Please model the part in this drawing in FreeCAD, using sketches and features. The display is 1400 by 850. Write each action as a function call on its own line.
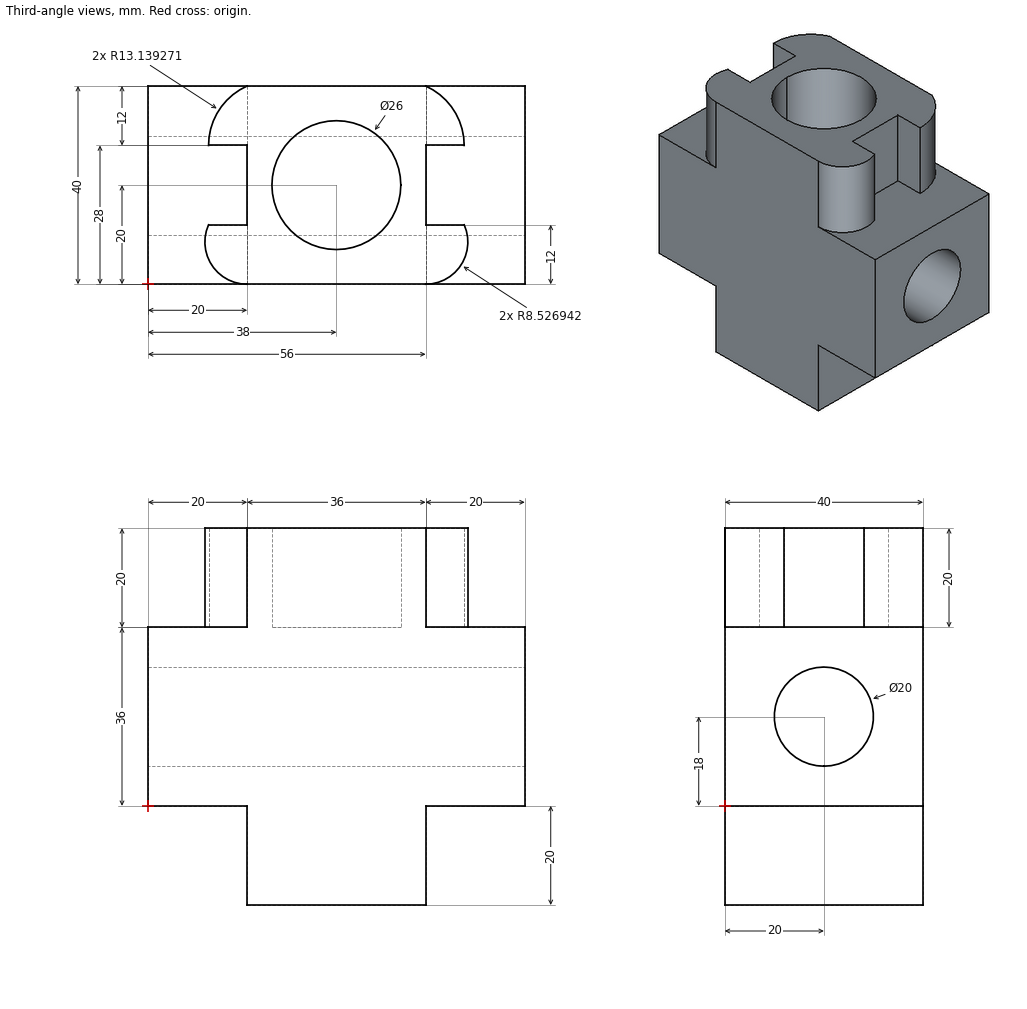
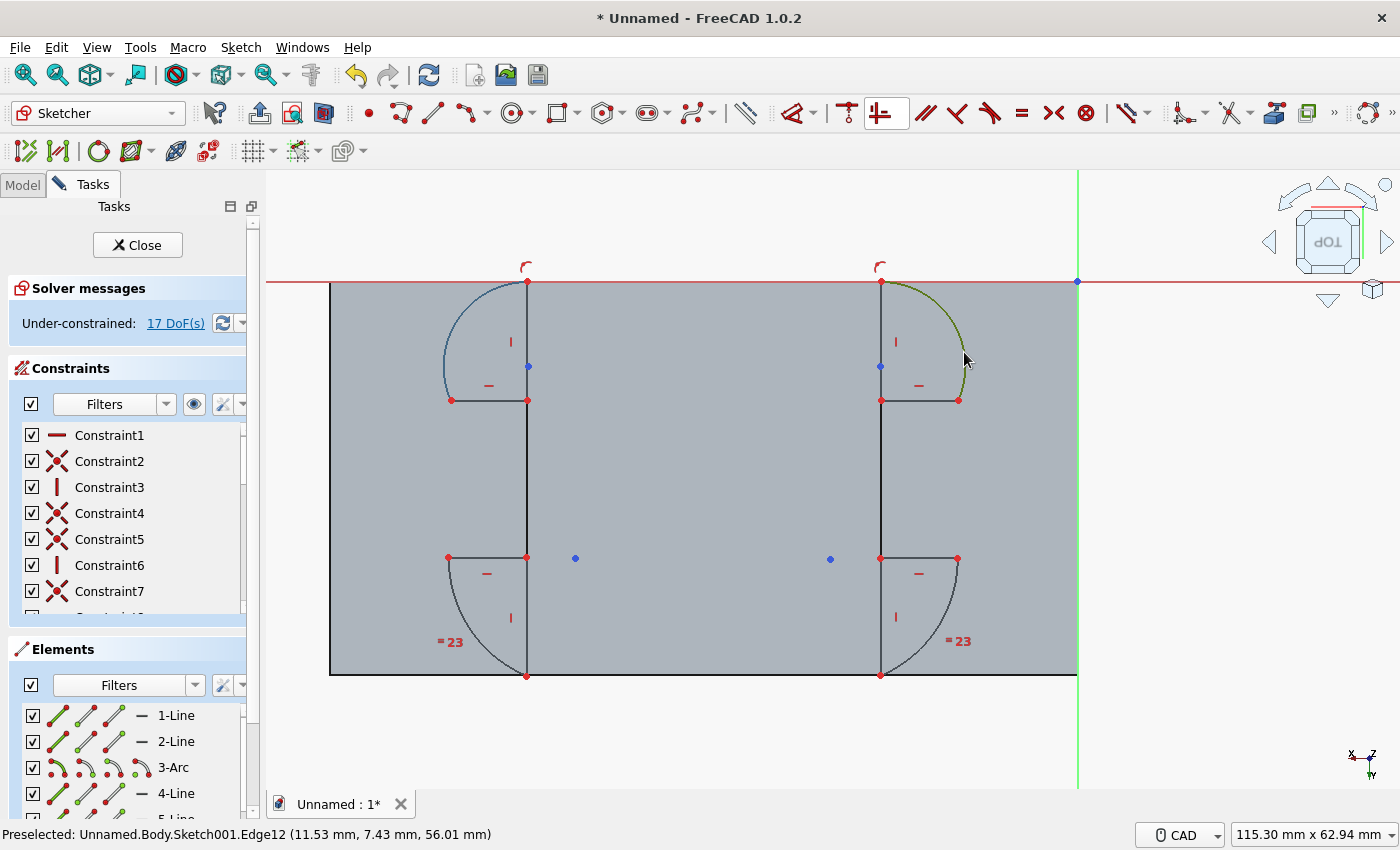
click(1022, 114)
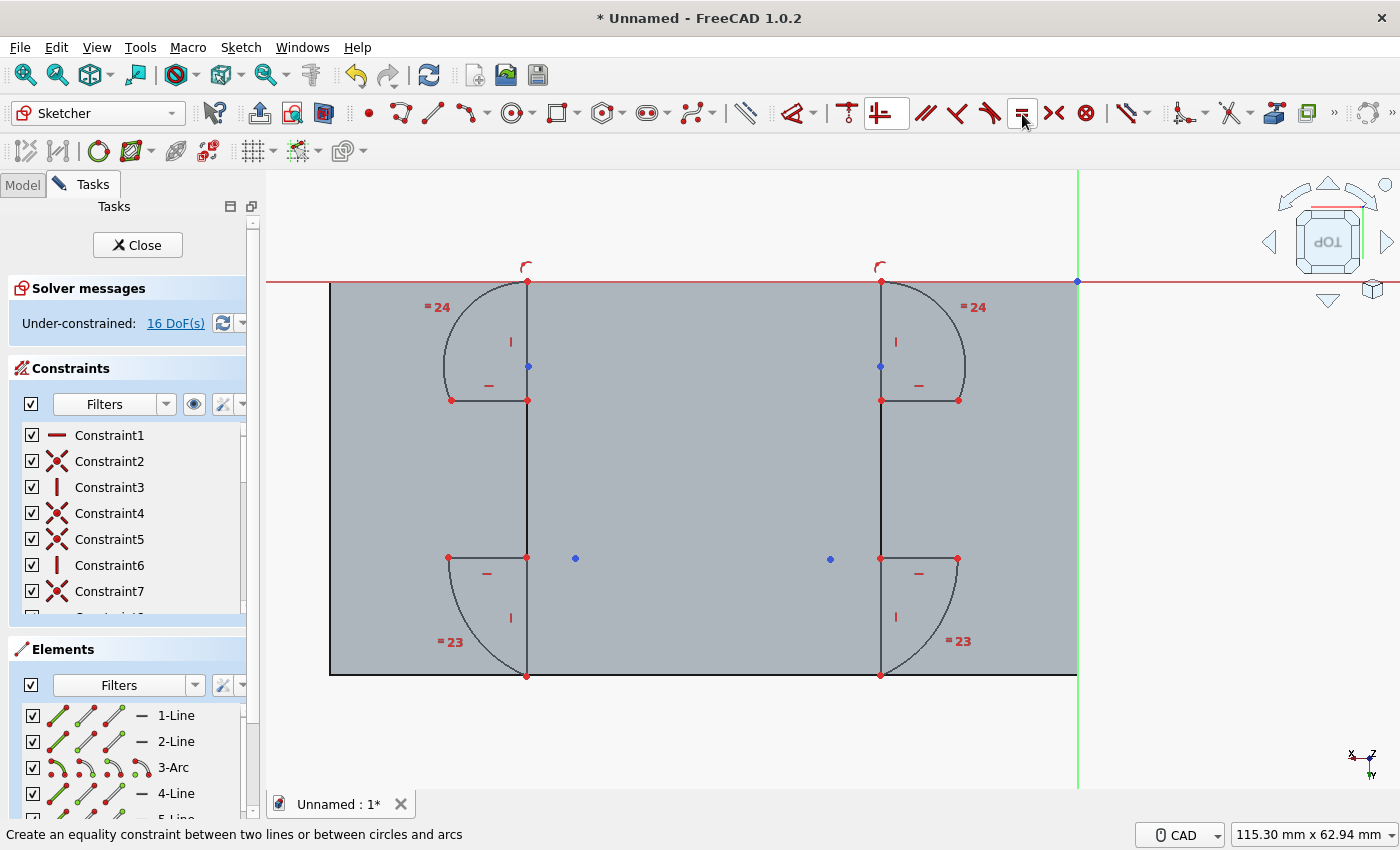
click(792, 114)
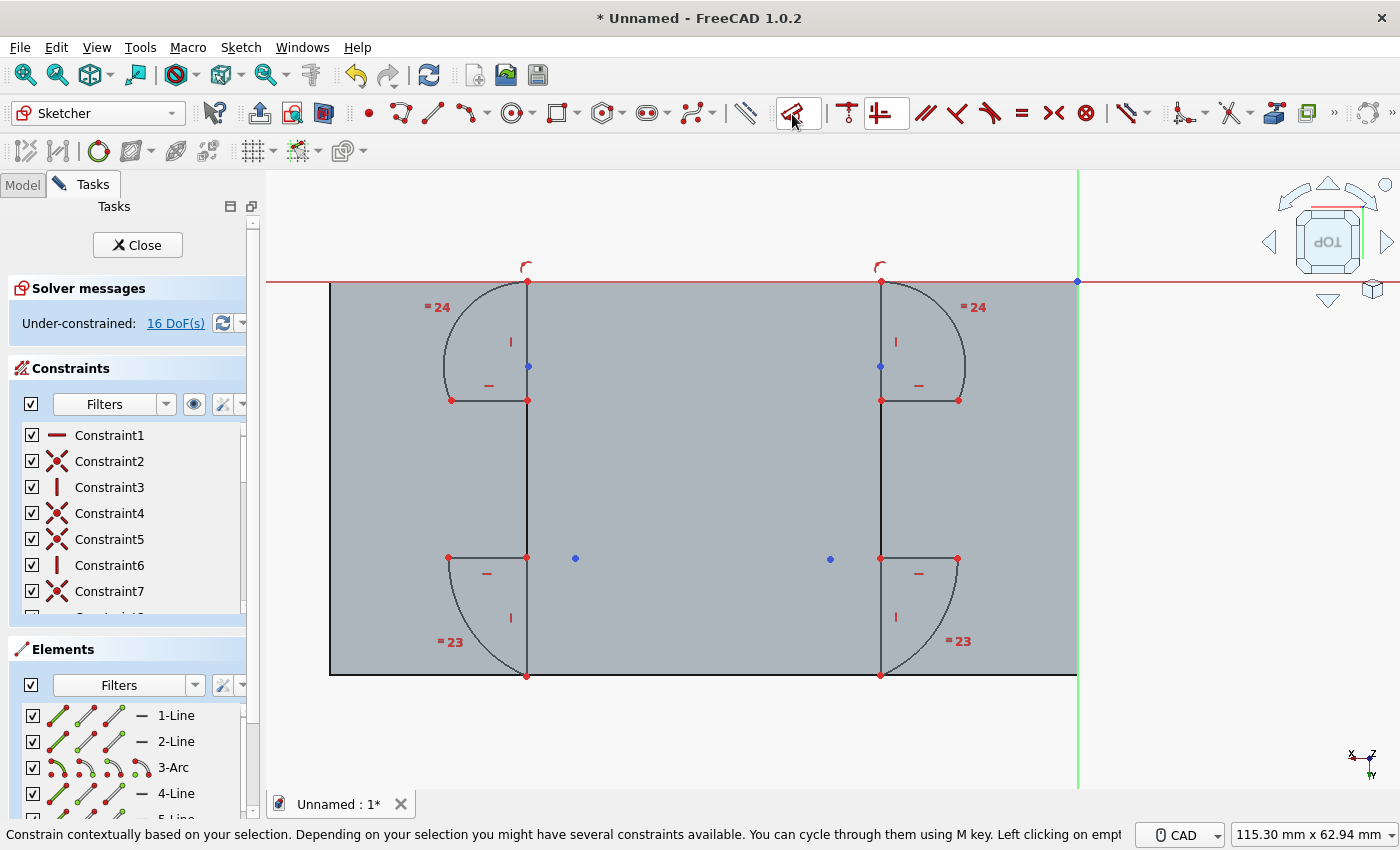
click(918, 651)
click(940, 674)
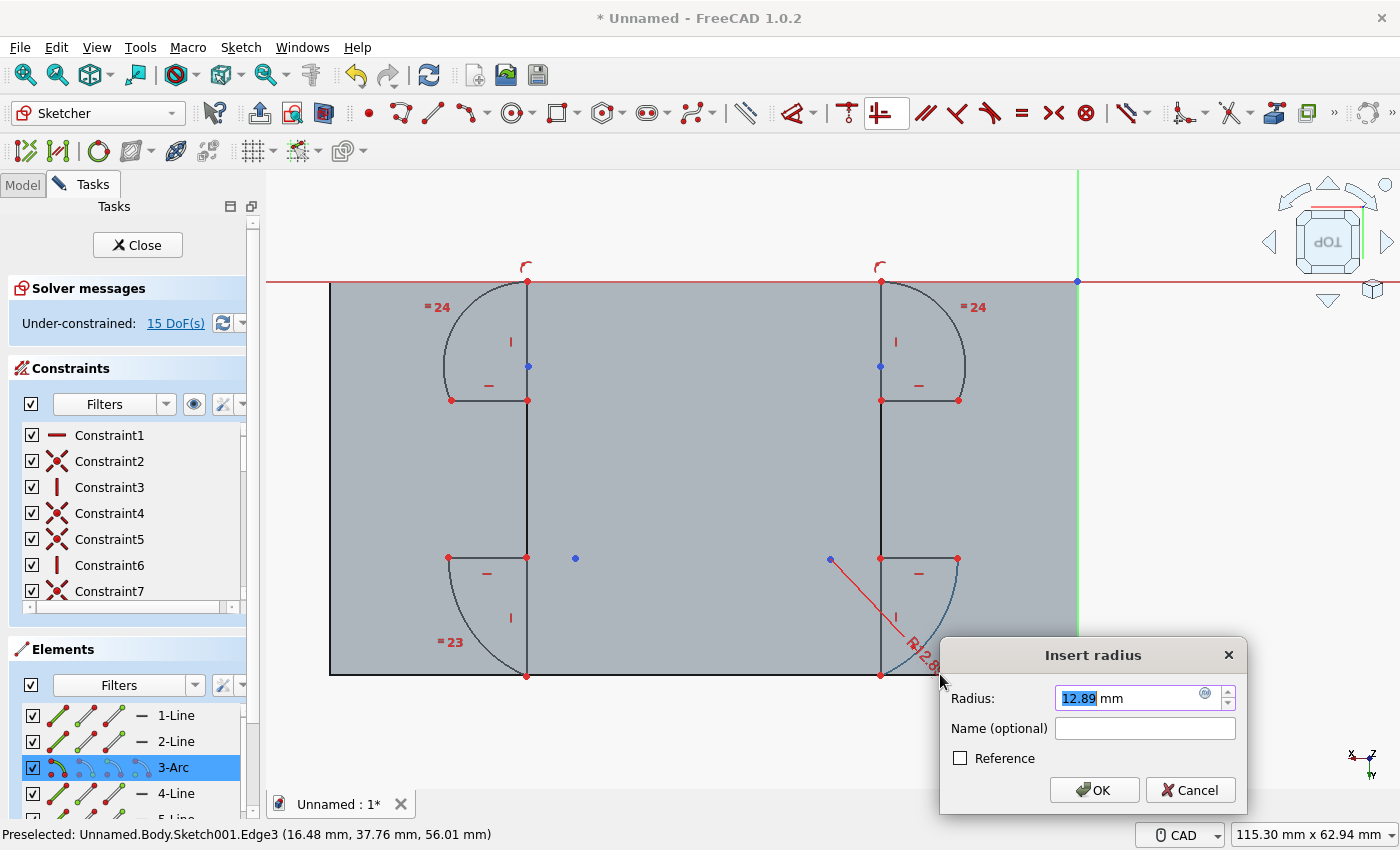
text(13.139271)
key(Return)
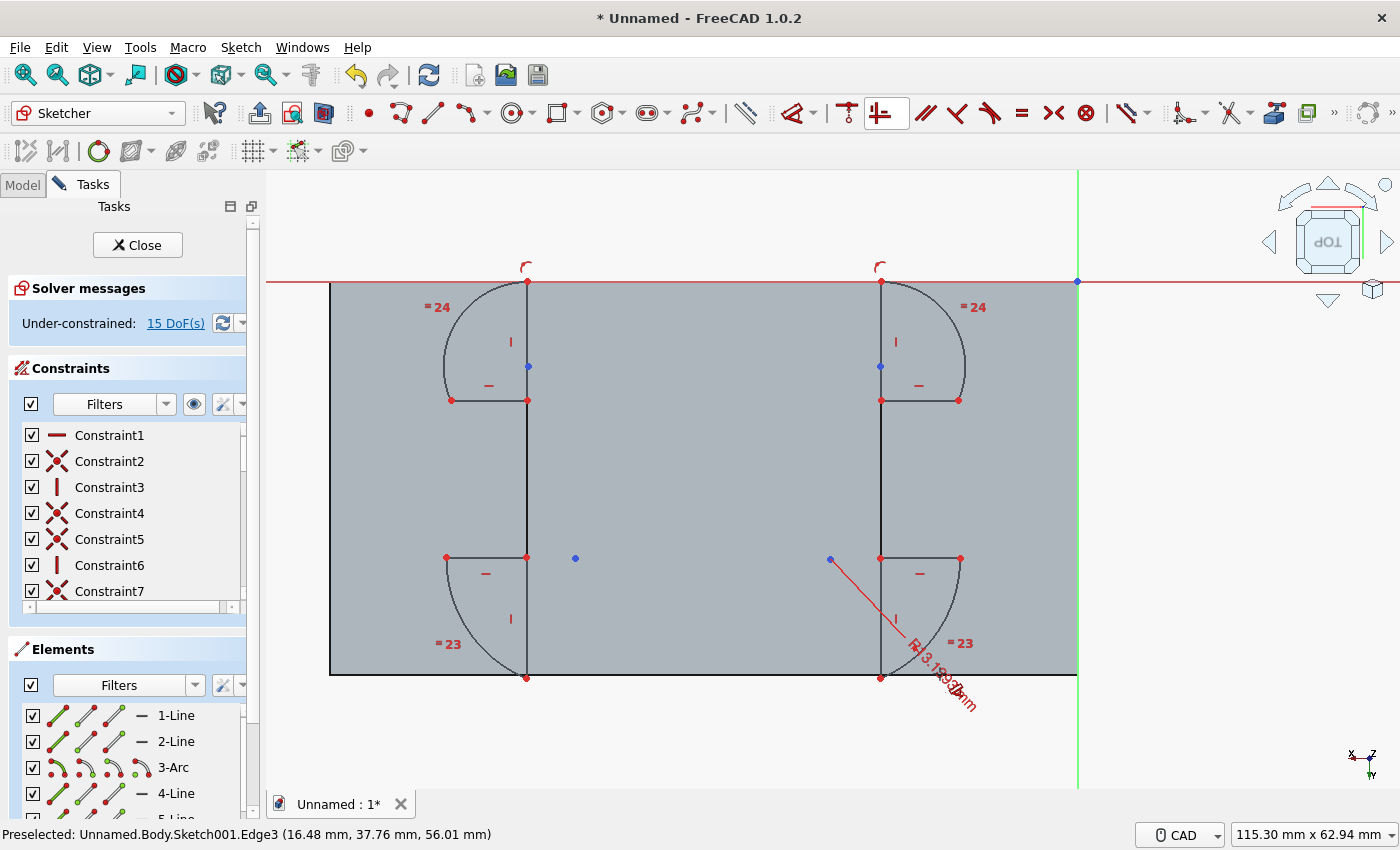
click(480, 297)
click(516, 251)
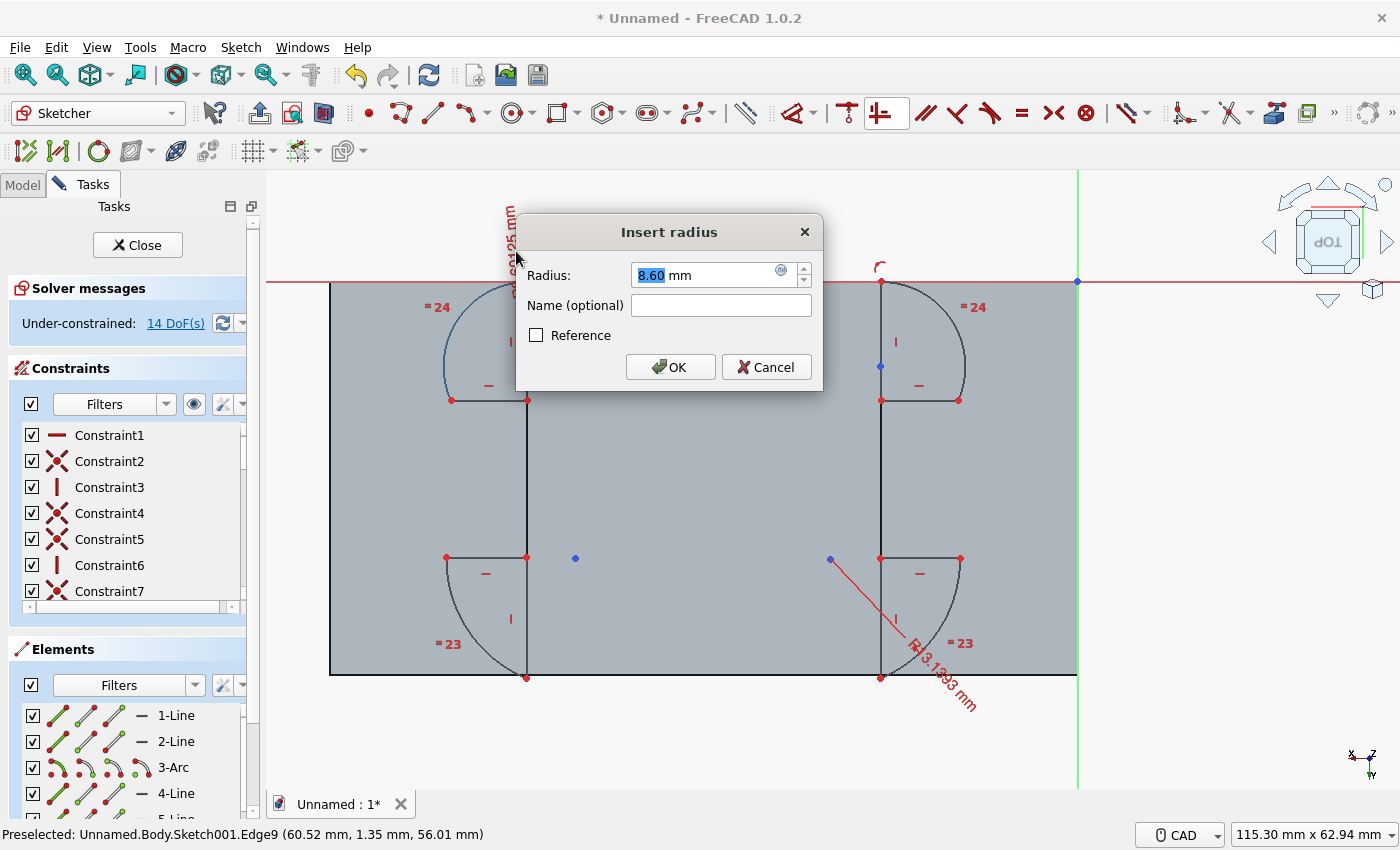
text(8.526942)
key(Return)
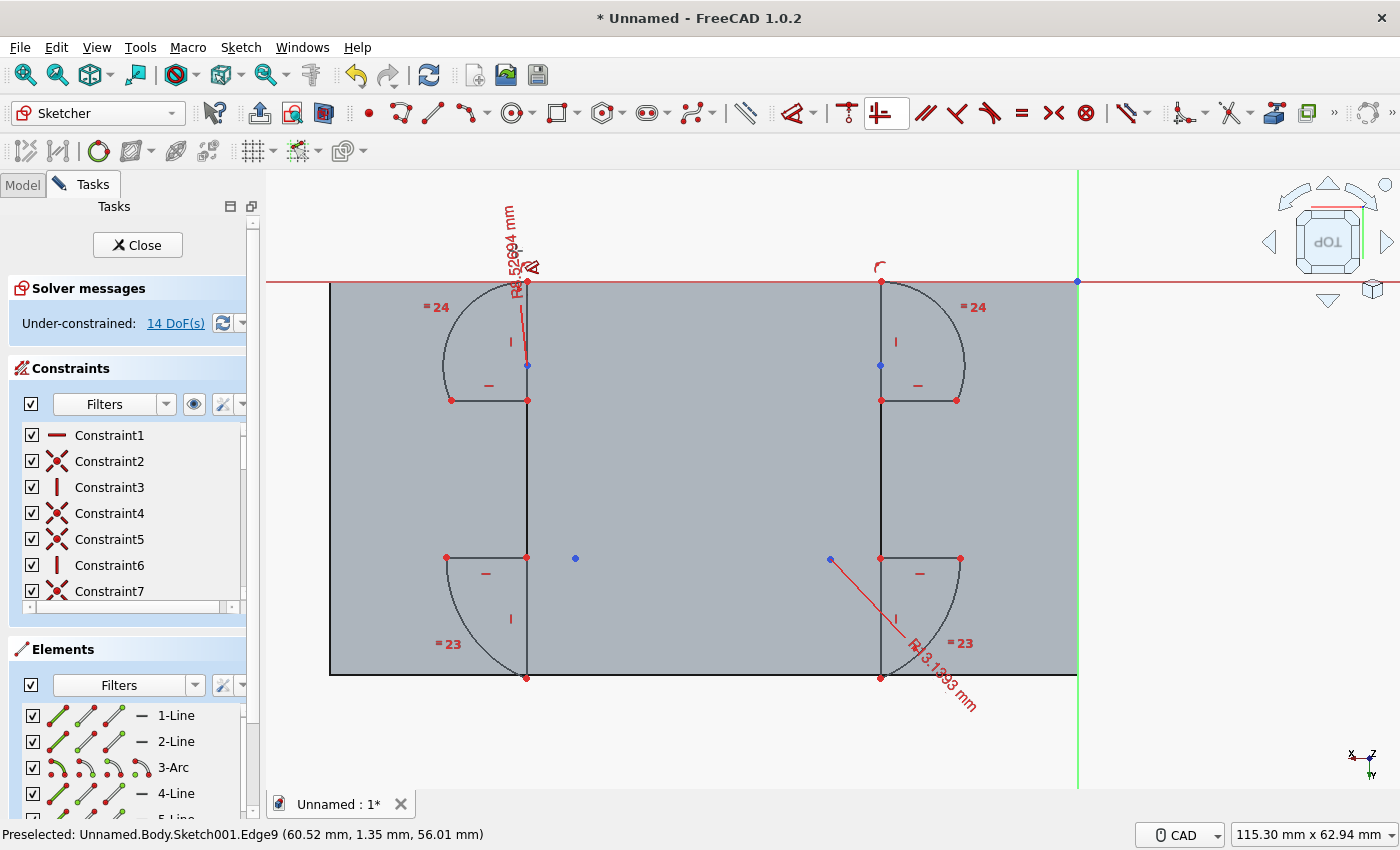
click(881, 594)
click(915, 618)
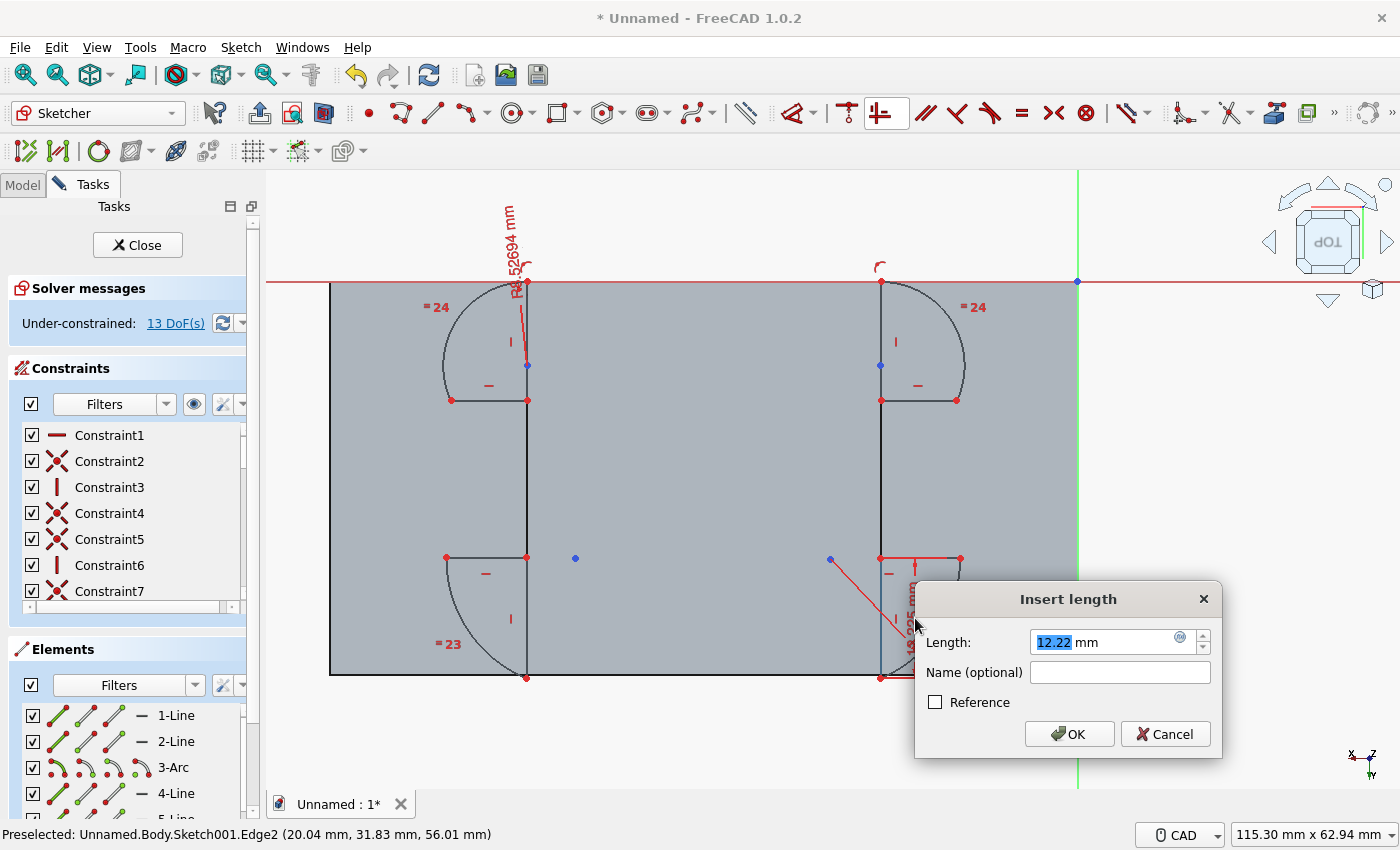
text(12)
key(Return)